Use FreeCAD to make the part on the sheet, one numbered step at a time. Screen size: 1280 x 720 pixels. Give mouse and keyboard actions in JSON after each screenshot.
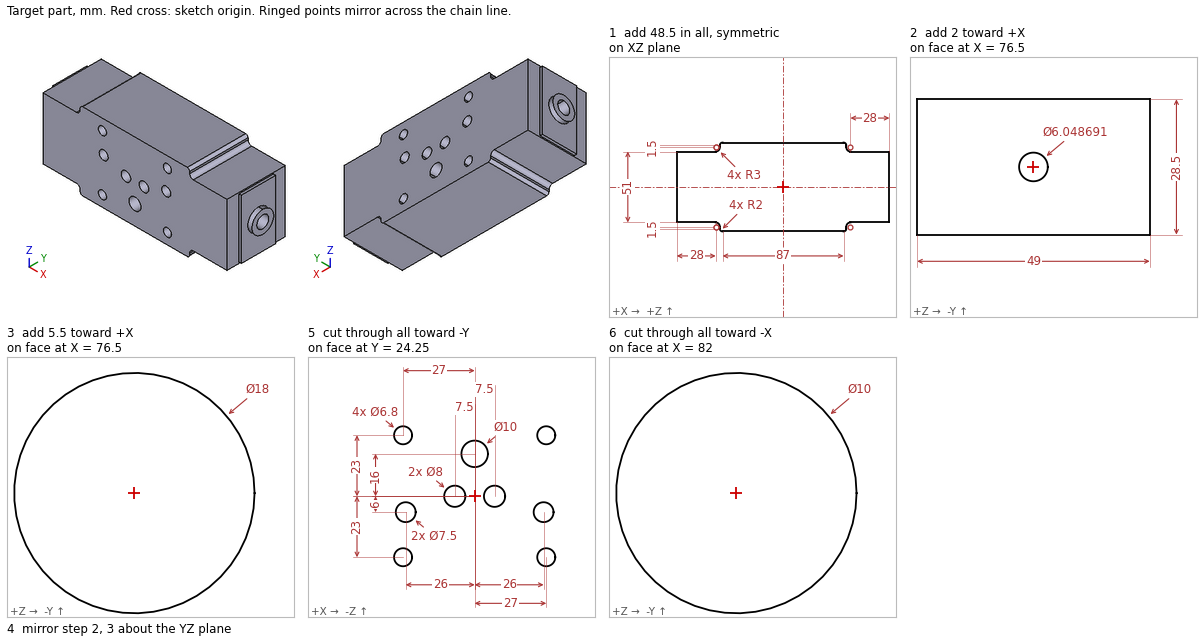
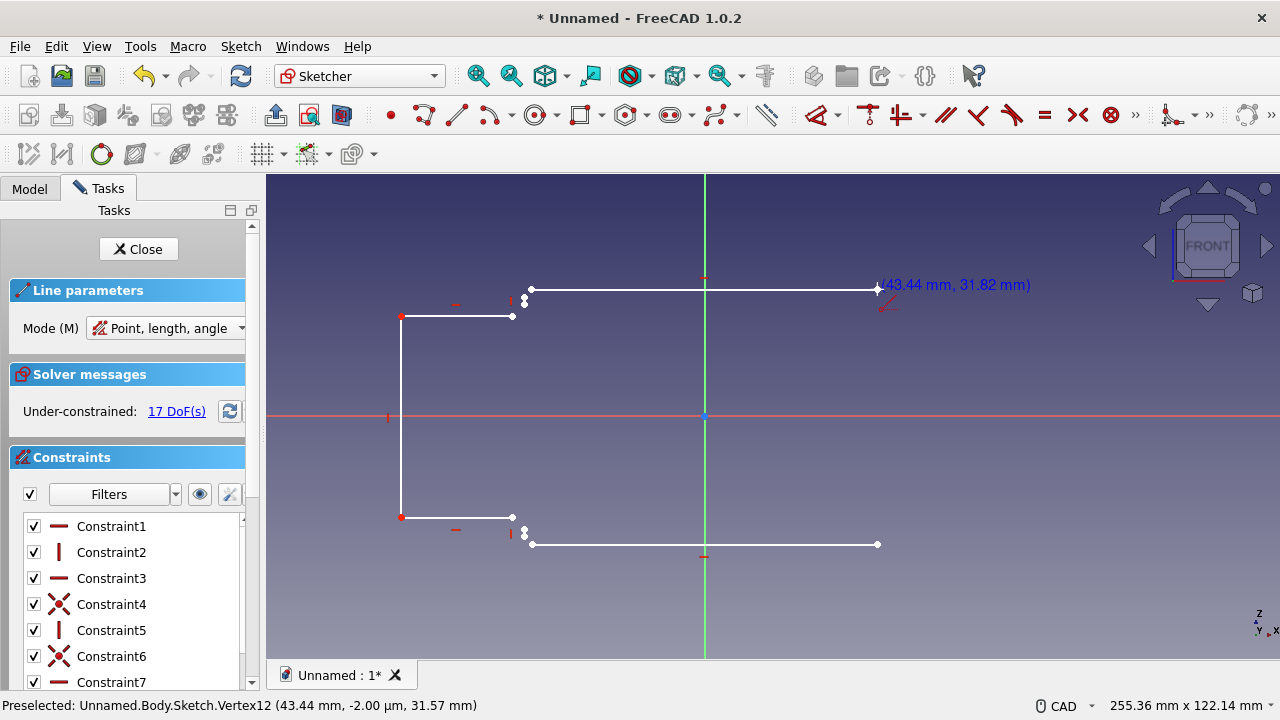
{"action": "scroll", "coordinate": [885, 297], "scroll_direction": "up", "scroll_amount": 2}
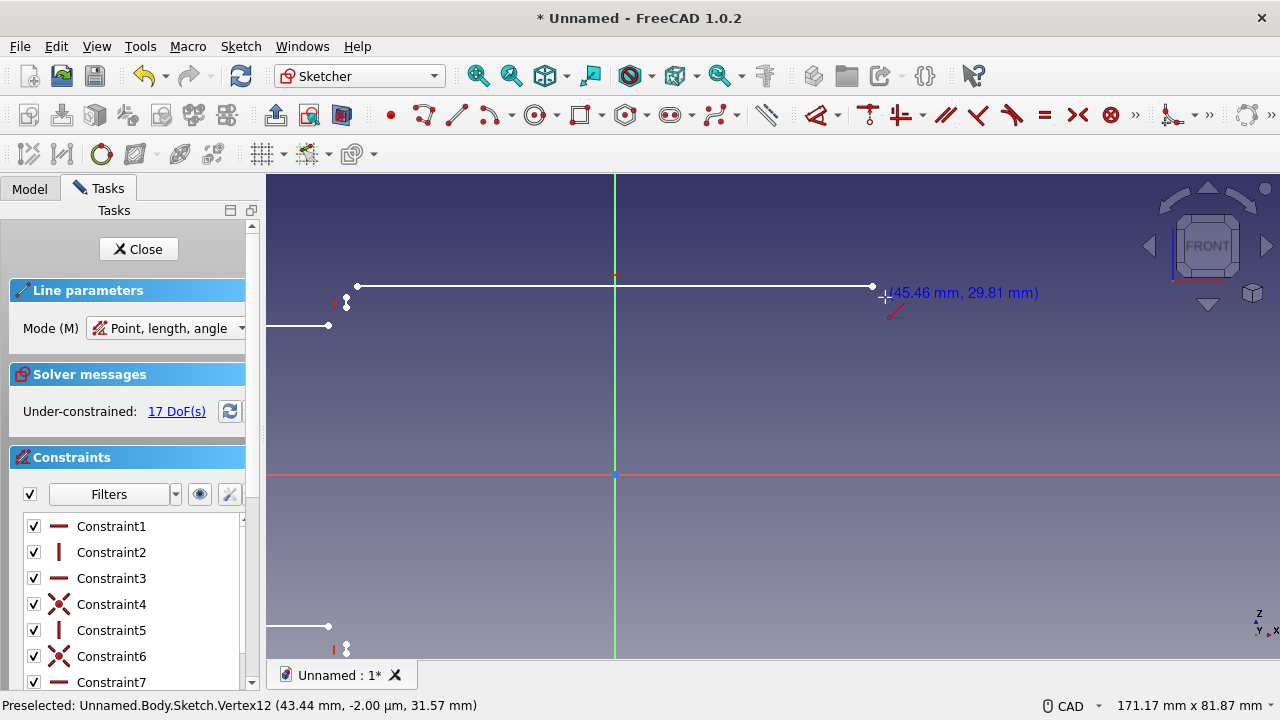
{"action": "left_click", "coordinate": [885, 297]}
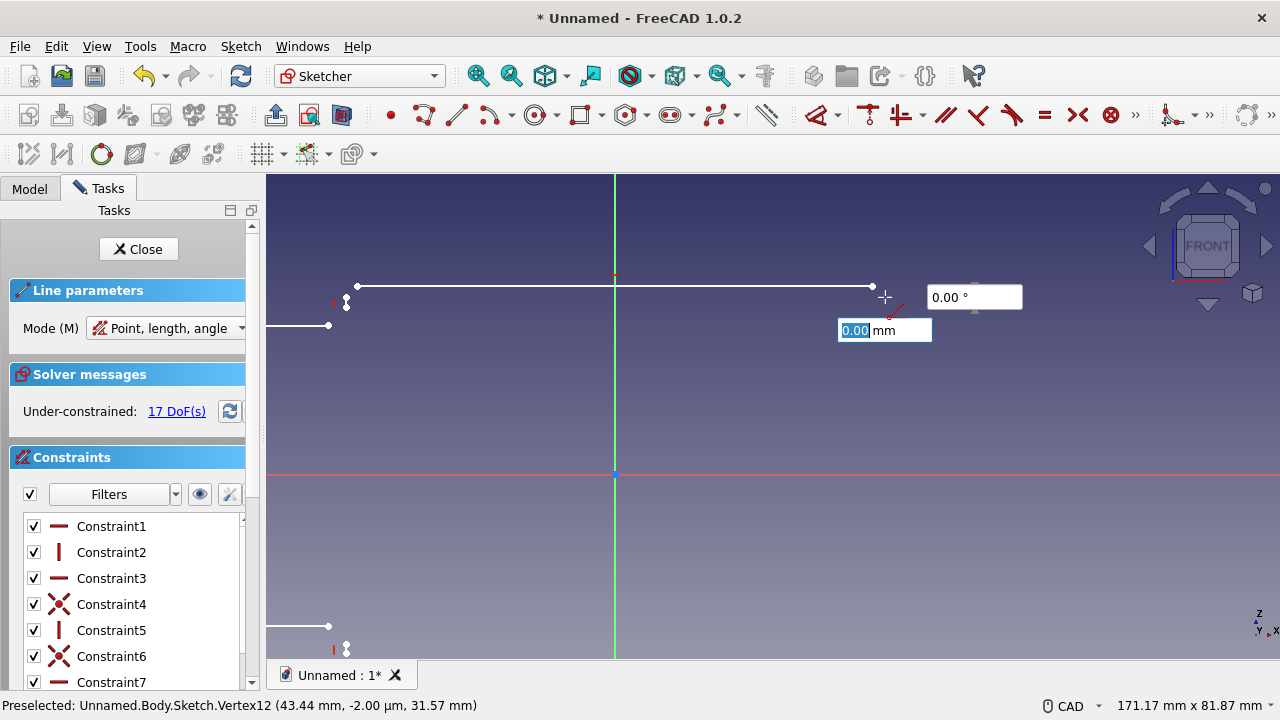
{"action": "scroll", "coordinate": [885, 306], "scroll_direction": "up", "scroll_amount": 3}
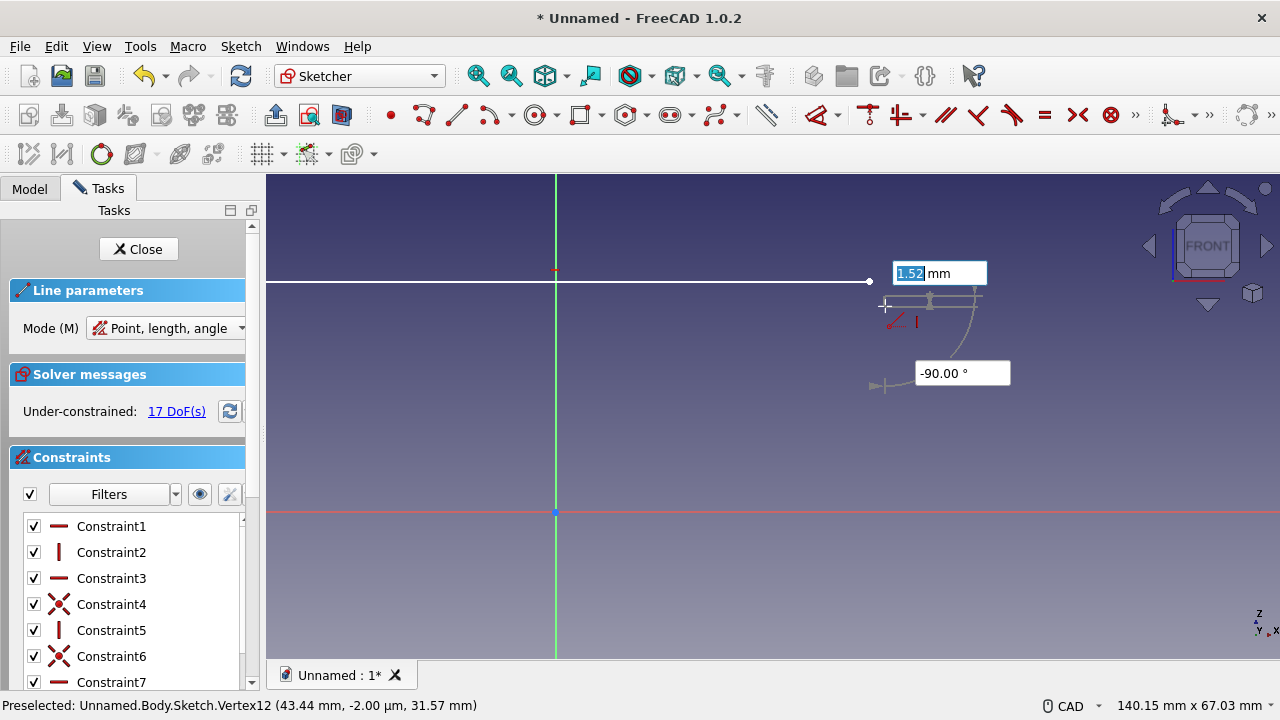
{"action": "left_click", "coordinate": [884, 306]}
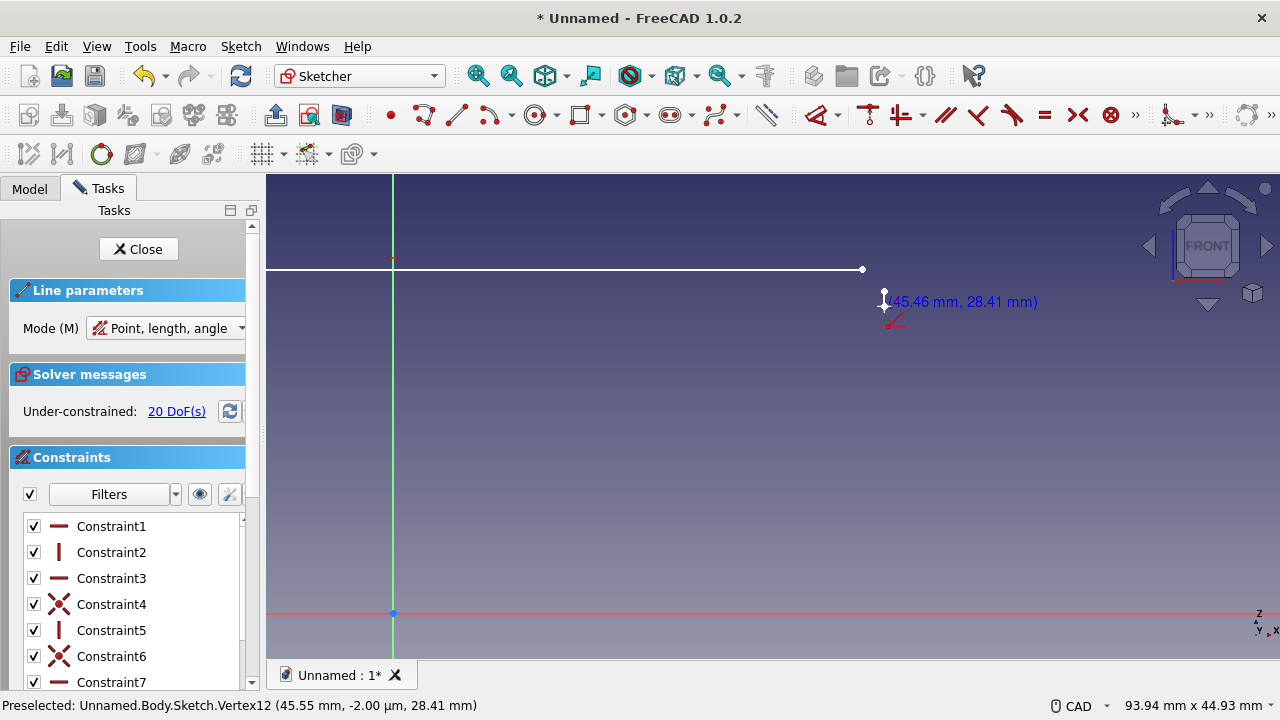
{"action": "left_click", "coordinate": [424, 116]}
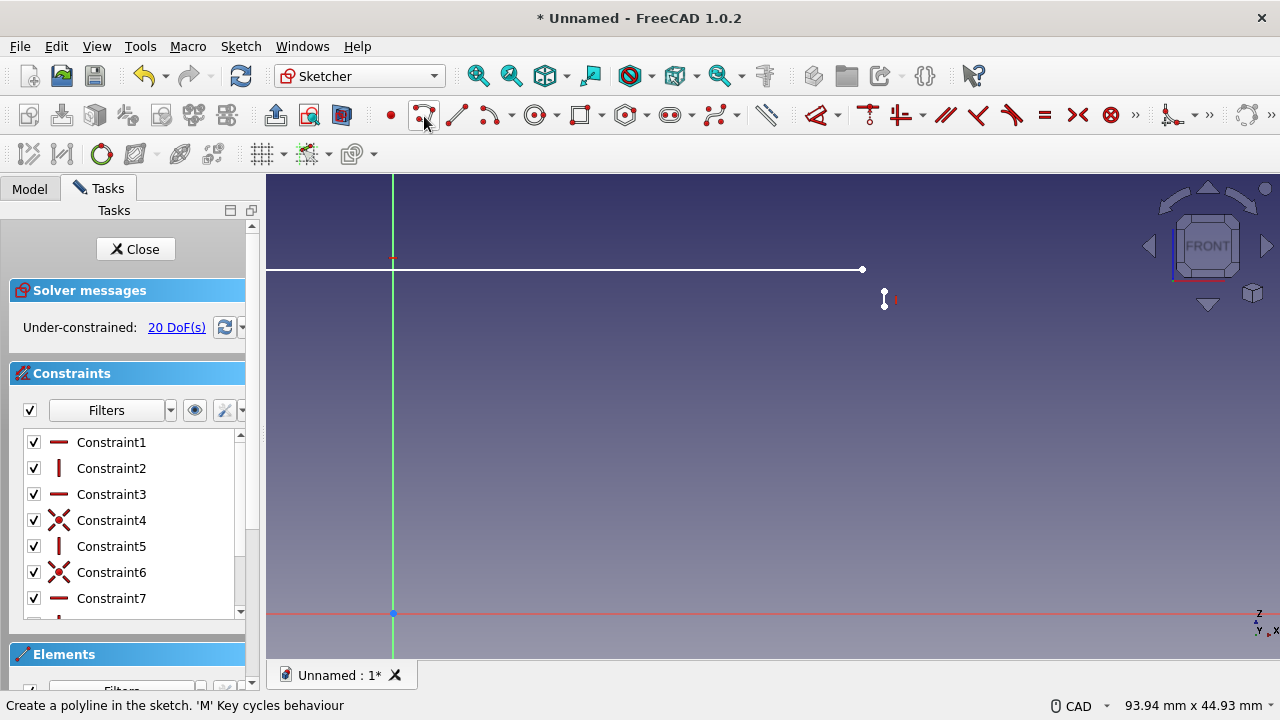
{"action": "left_click", "coordinate": [917, 338]}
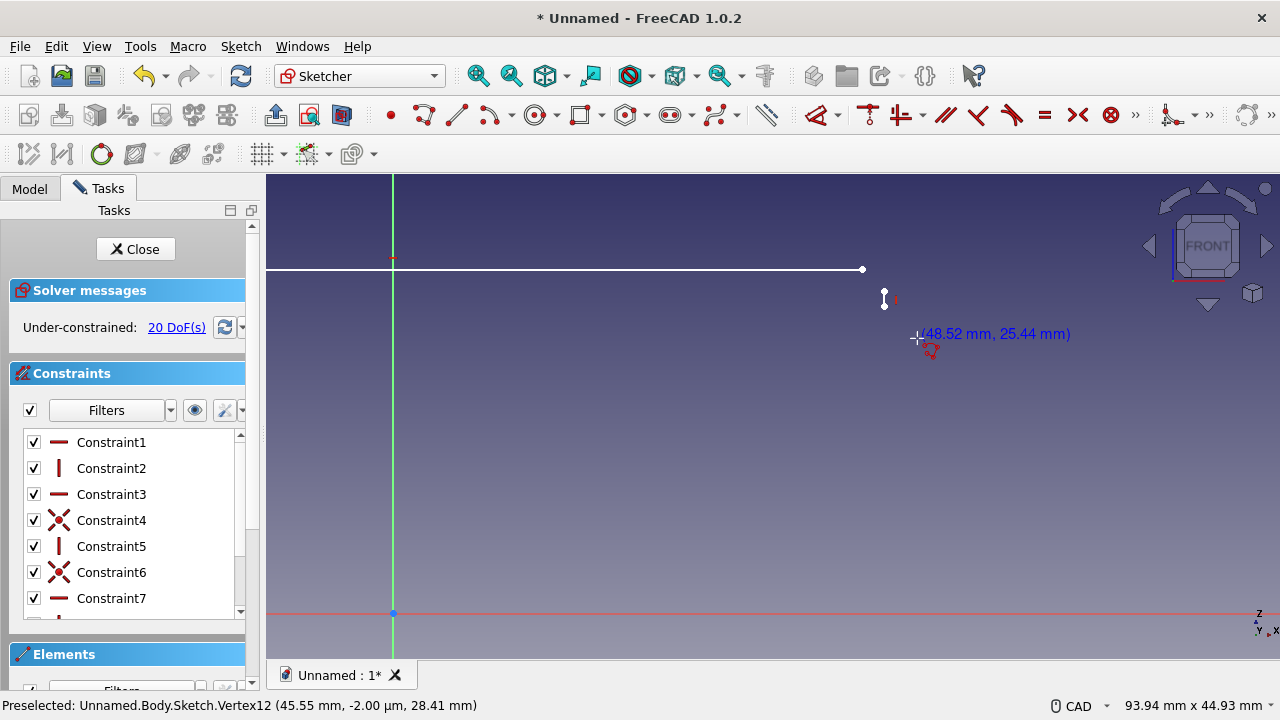
{"action": "scroll", "coordinate": [886, 302], "scroll_direction": "down", "scroll_amount": 5}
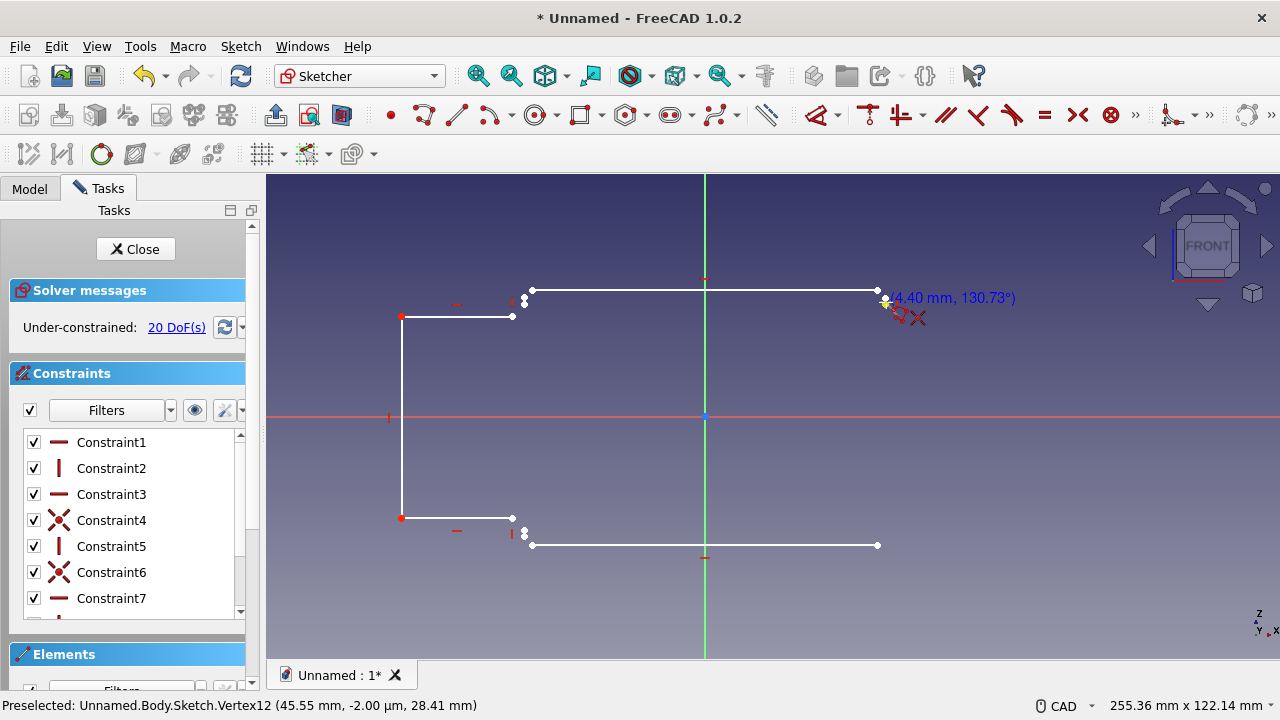
{"action": "left_click", "coordinate": [1009, 315]}
{"action": "left_click", "coordinate": [1009, 518]}
{"action": "left_click", "coordinate": [898, 518]}
{"action": "right_click", "coordinate": [898, 518]}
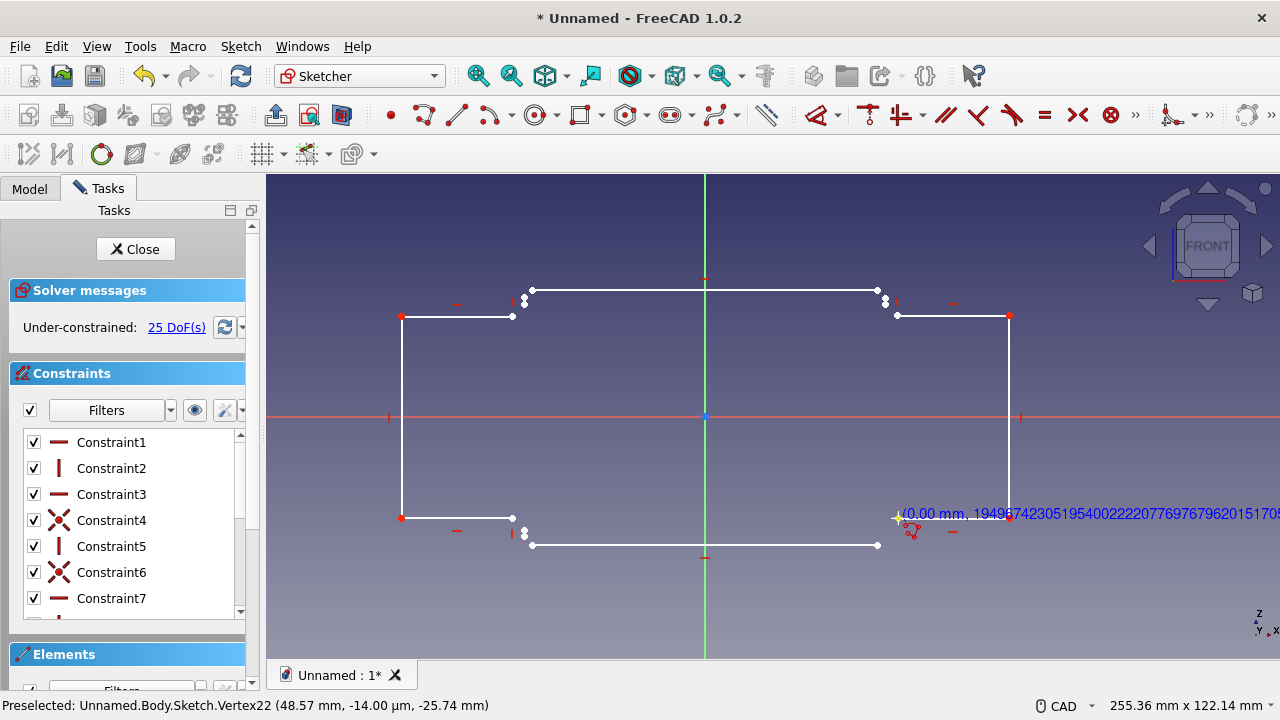
{"action": "left_click", "coordinate": [457, 116]}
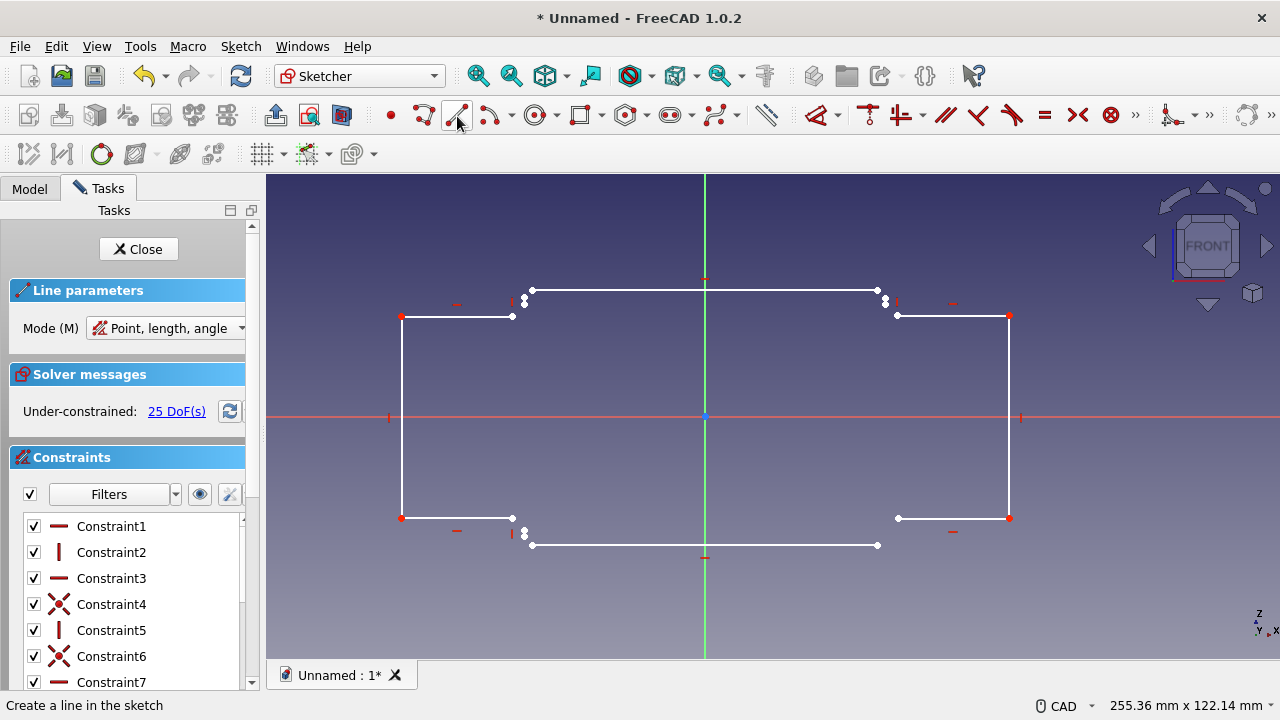
{"action": "left_click", "coordinate": [886, 530]}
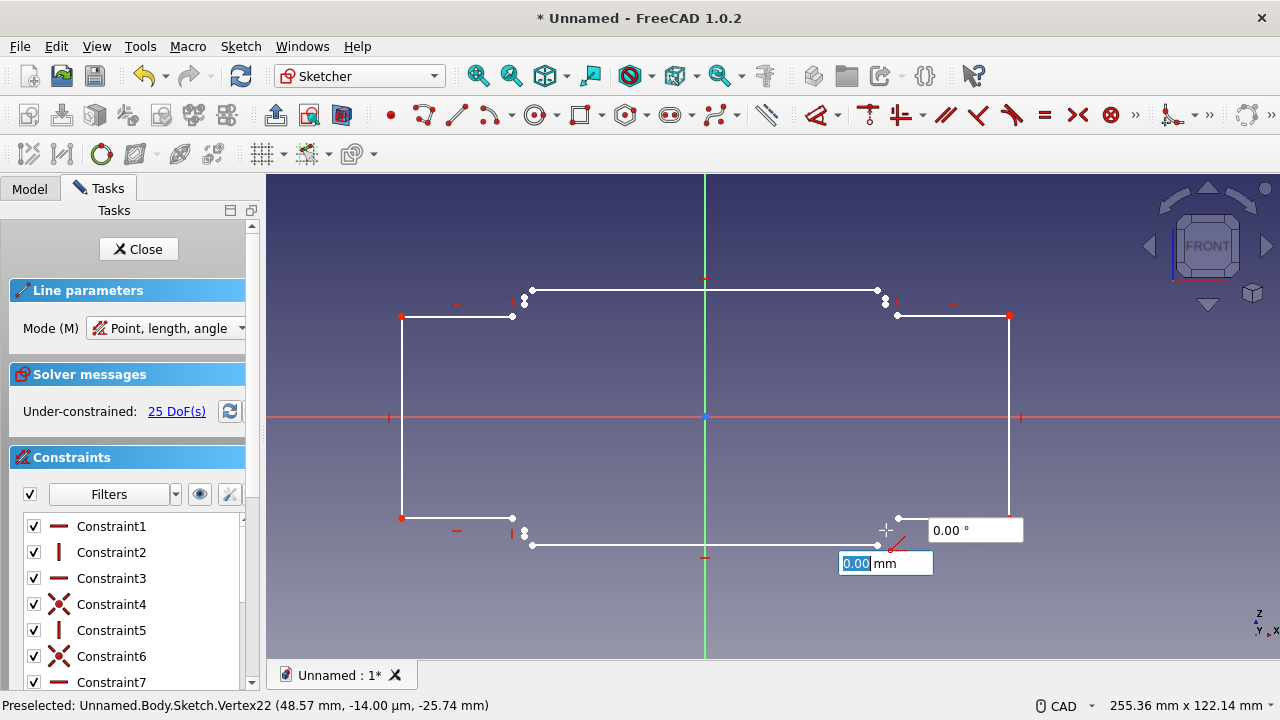
{"action": "scroll", "coordinate": [886, 536], "scroll_direction": "up", "scroll_amount": 5}